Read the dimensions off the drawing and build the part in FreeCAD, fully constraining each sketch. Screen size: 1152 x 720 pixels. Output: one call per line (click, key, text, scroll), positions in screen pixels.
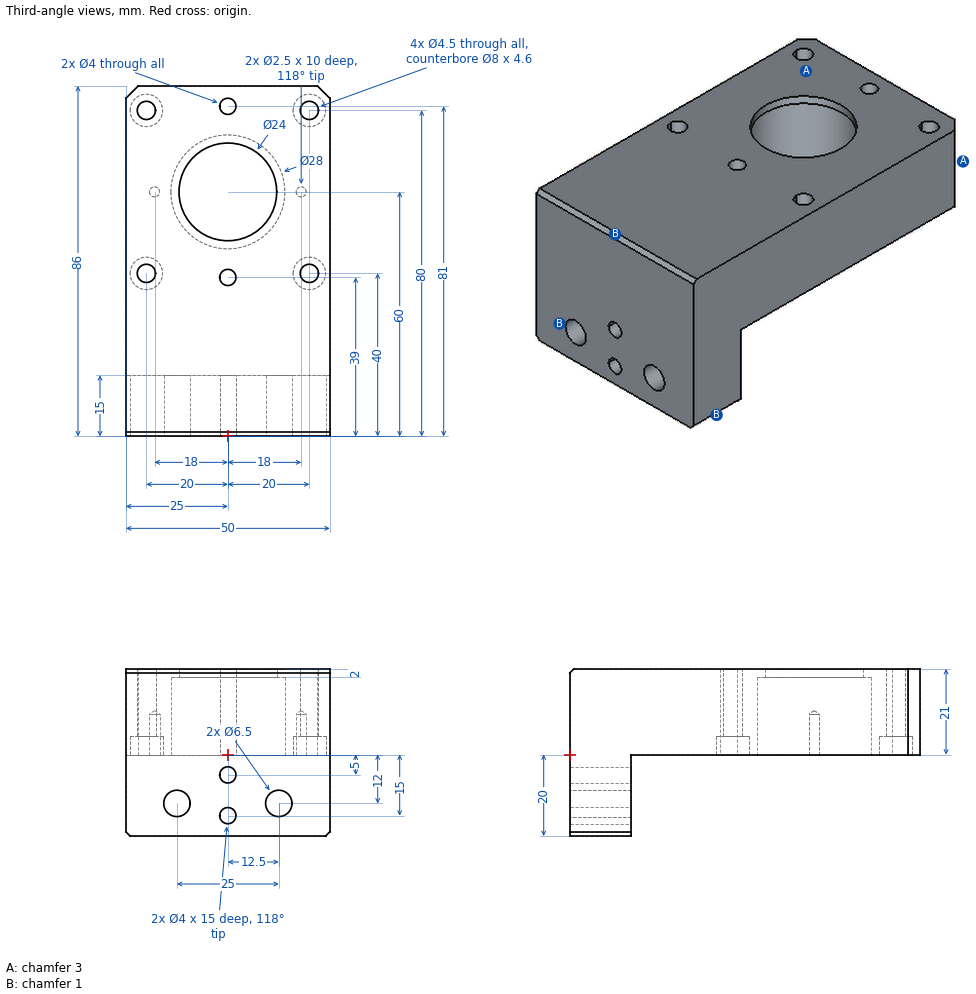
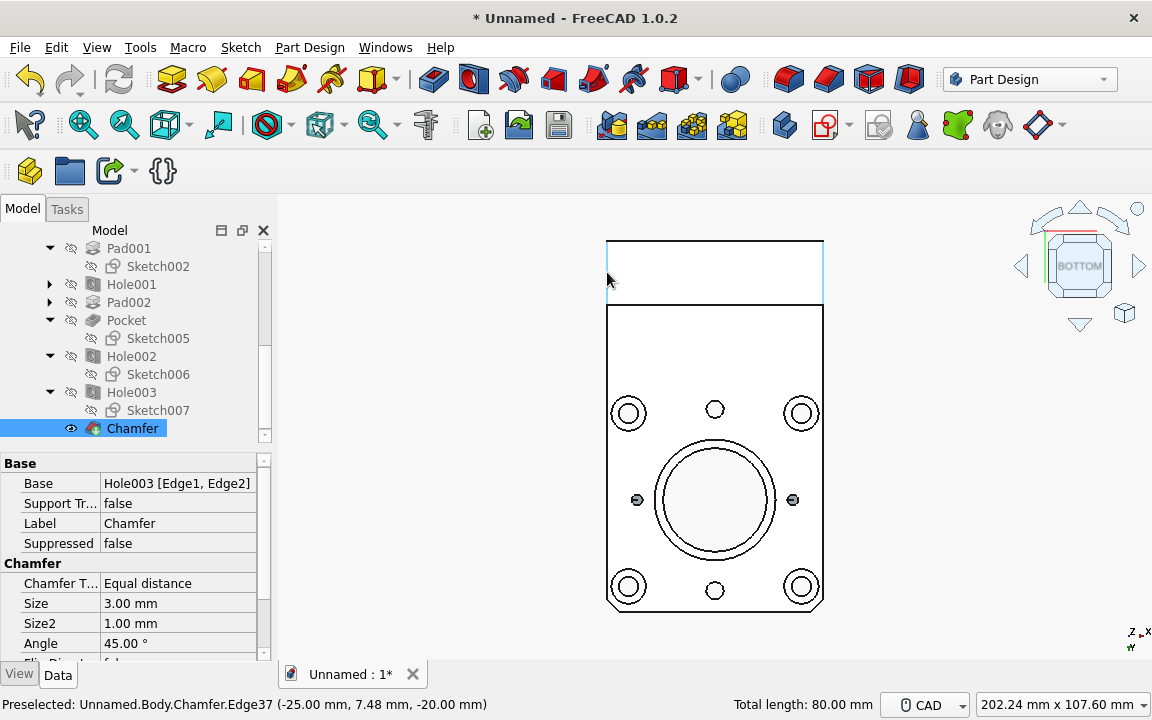
click(830, 80)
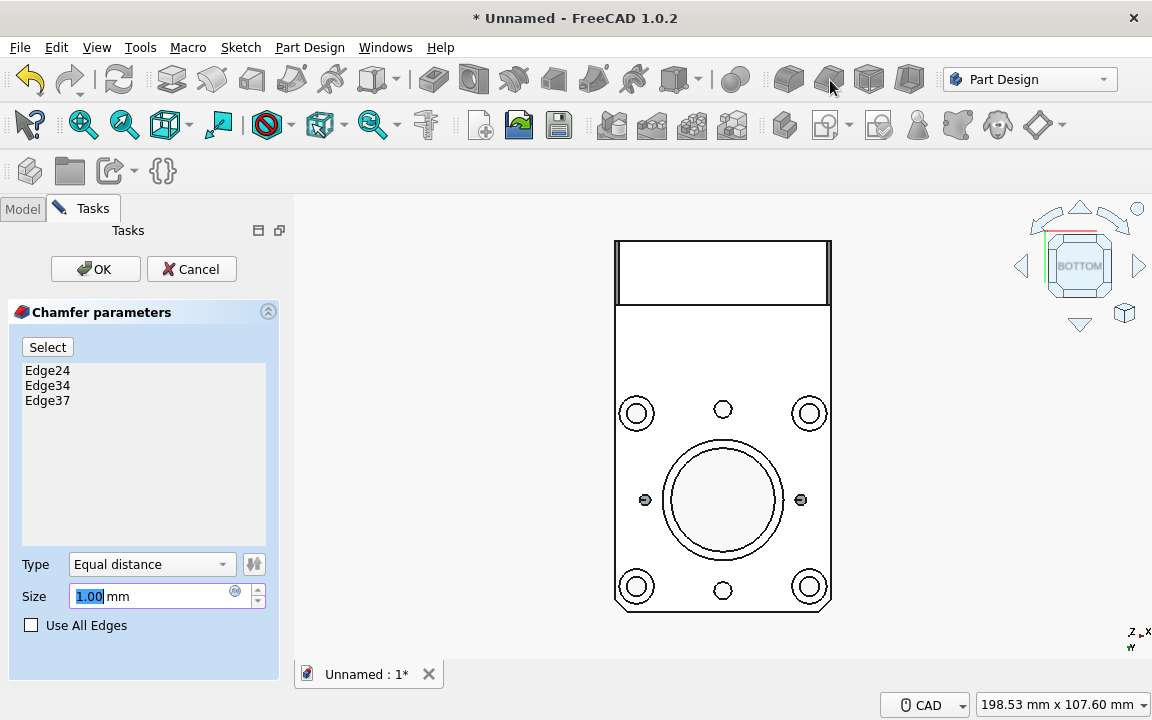
text(1)
key(Tab)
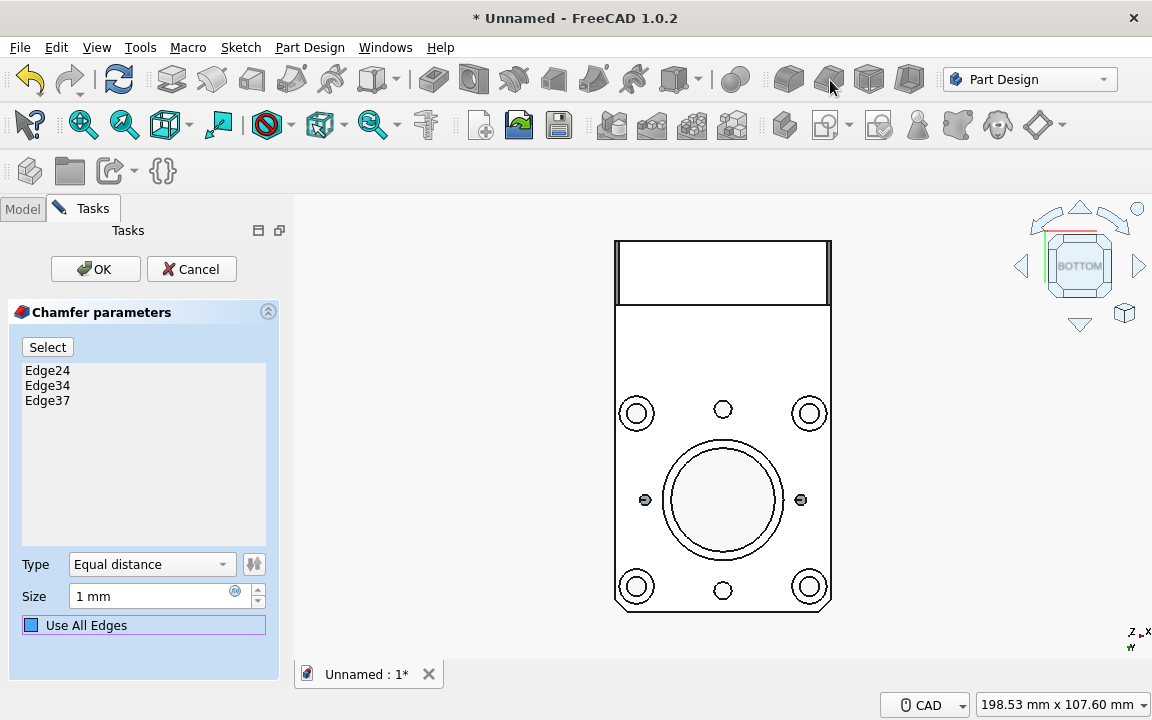
click(96, 269)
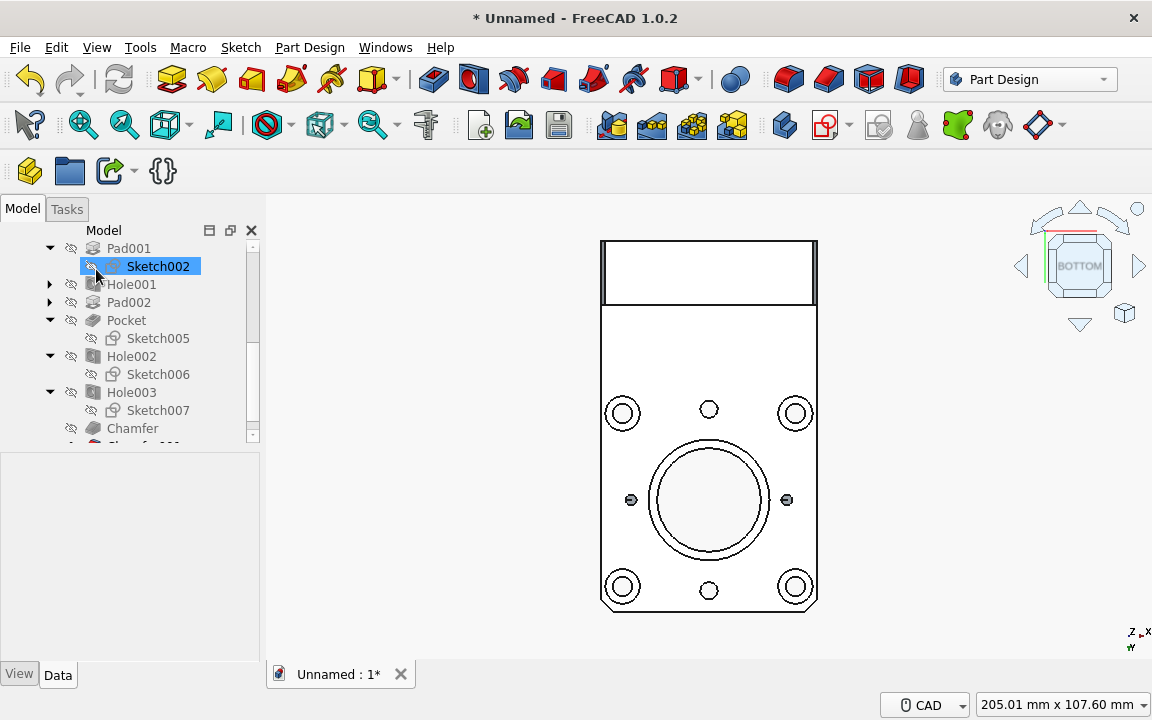
key(0)